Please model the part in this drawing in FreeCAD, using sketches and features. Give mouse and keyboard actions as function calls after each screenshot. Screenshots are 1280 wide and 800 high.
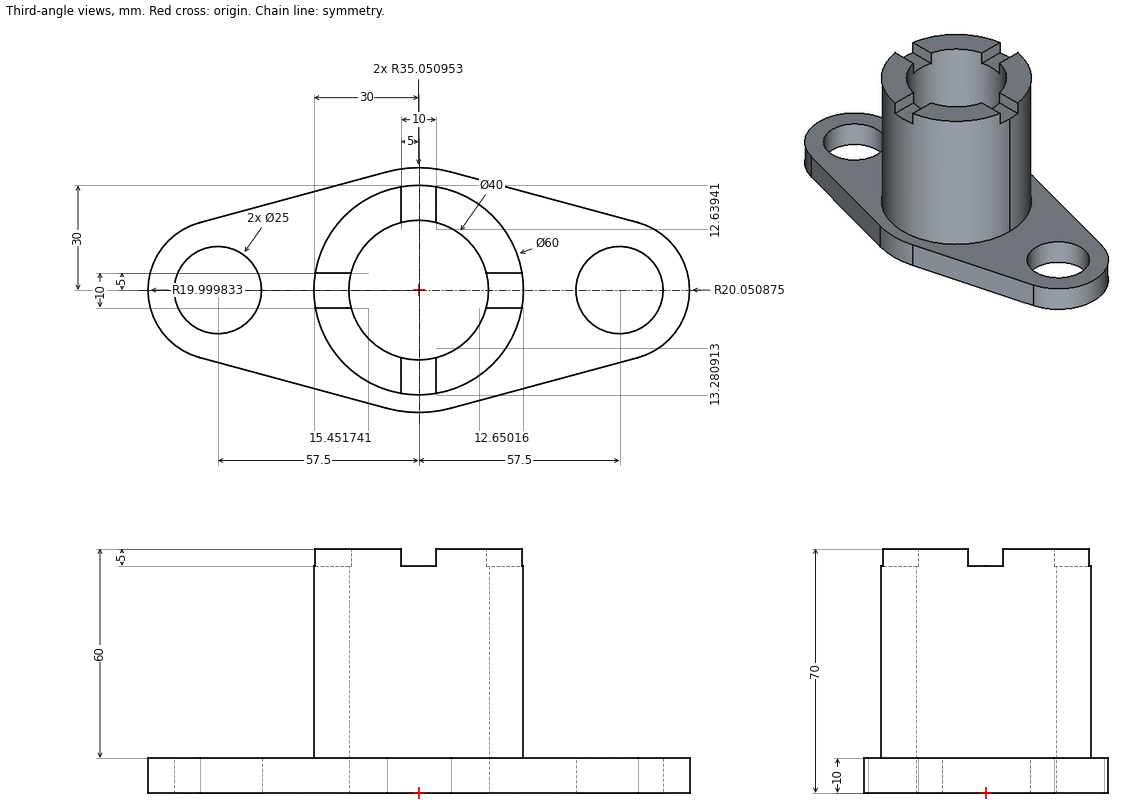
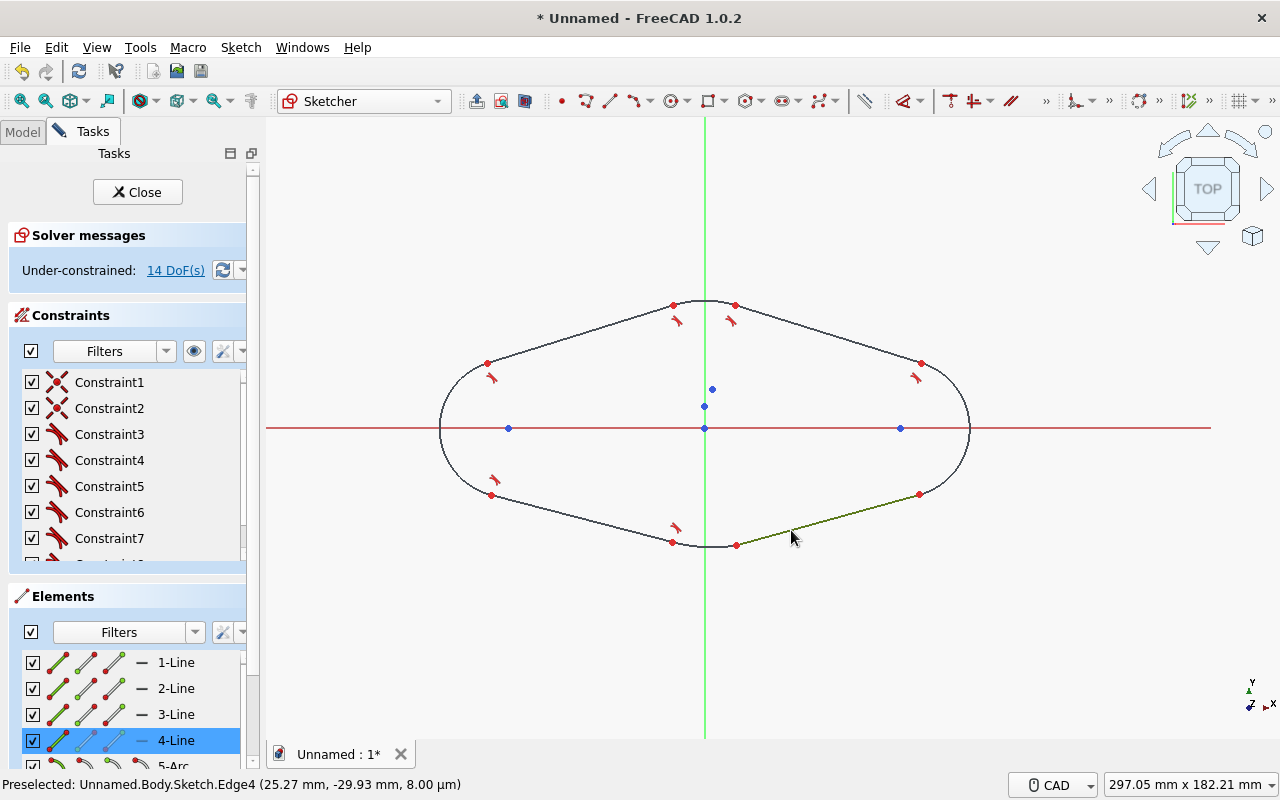
click(692, 546)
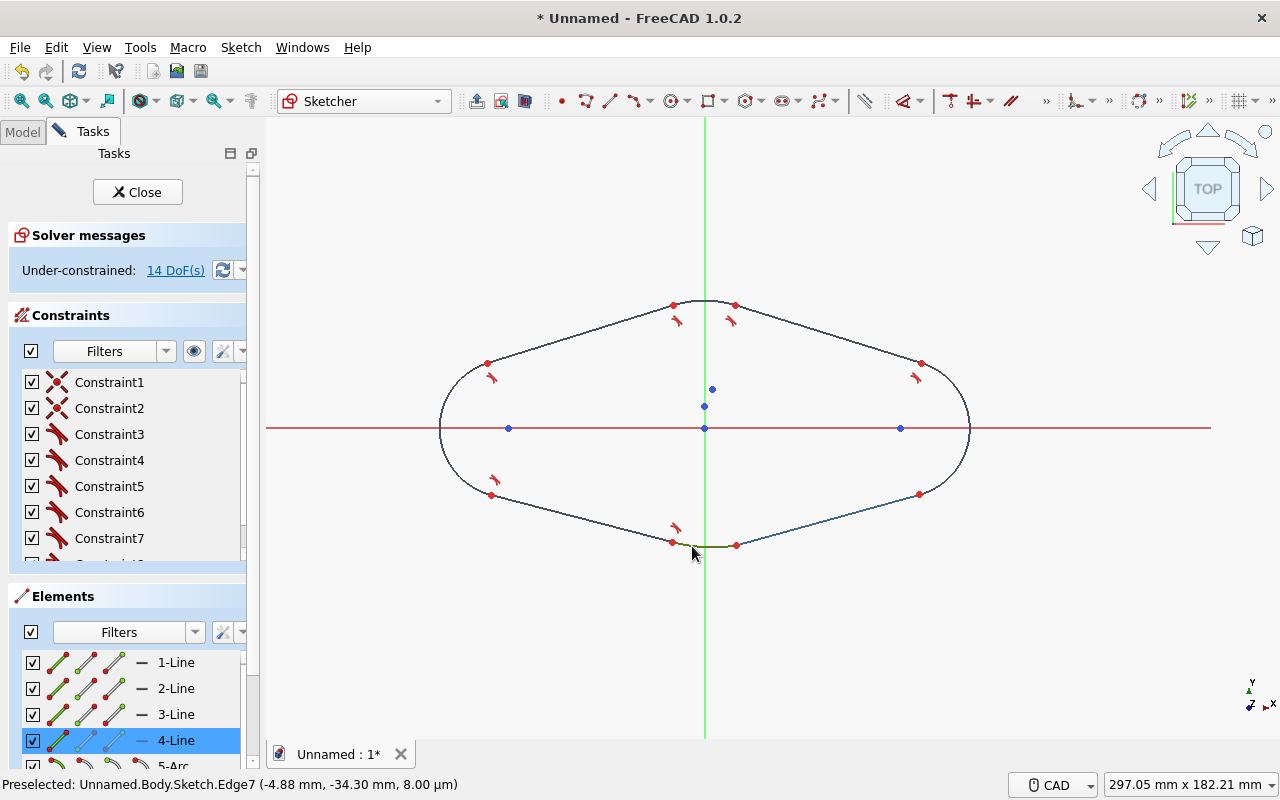
key(t)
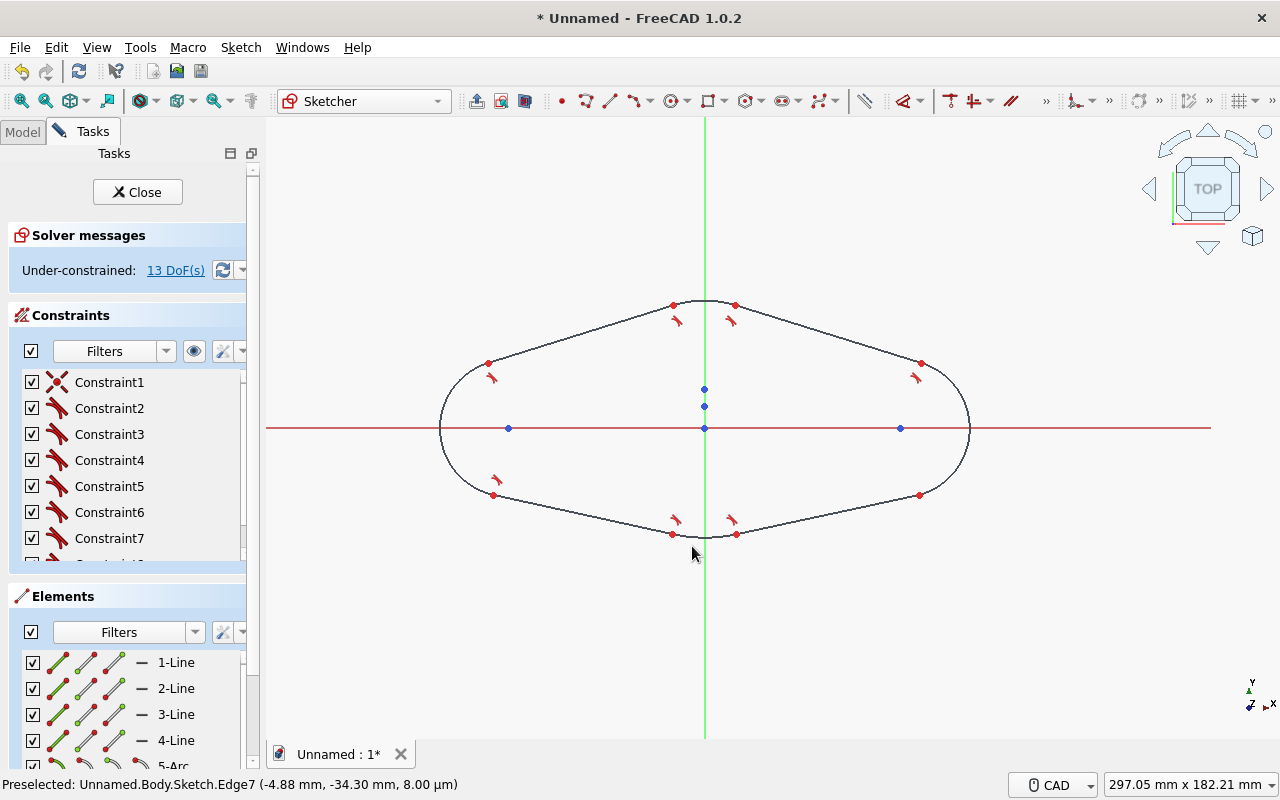
click(791, 523)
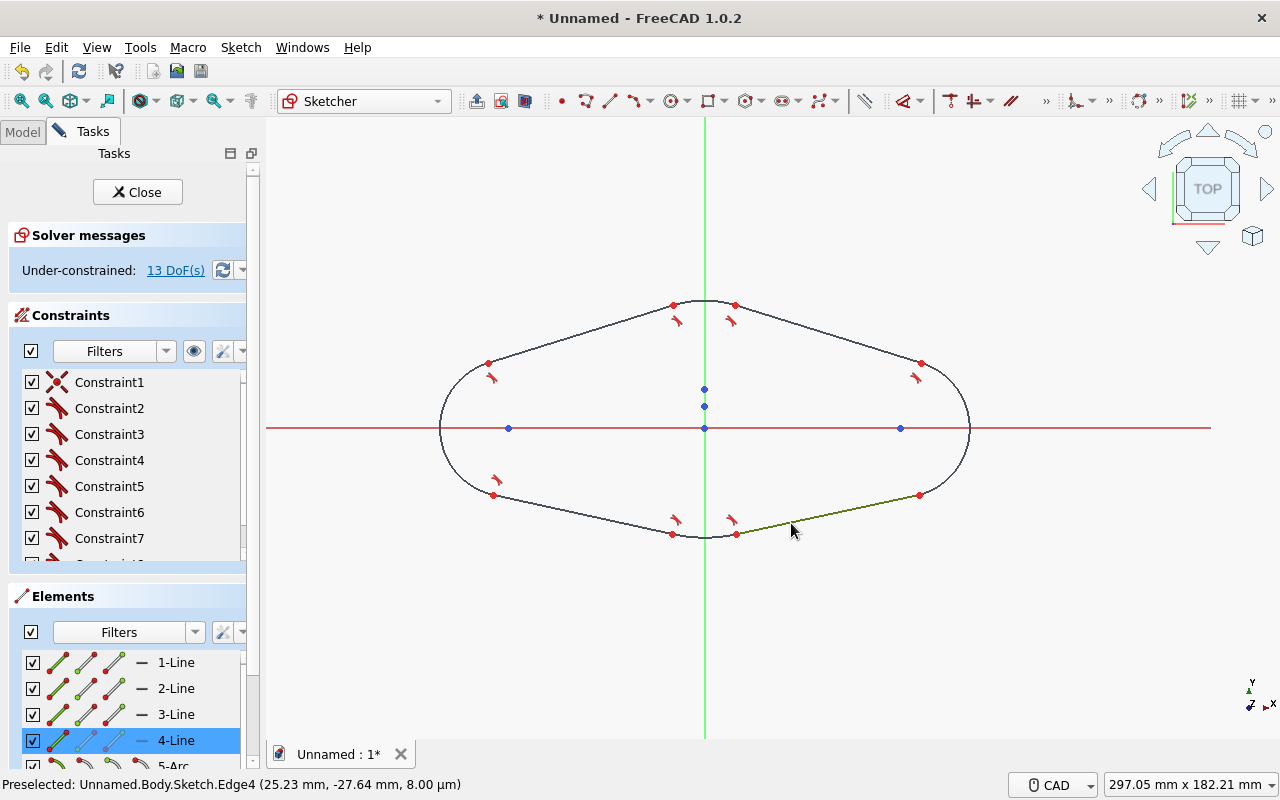
click(960, 464)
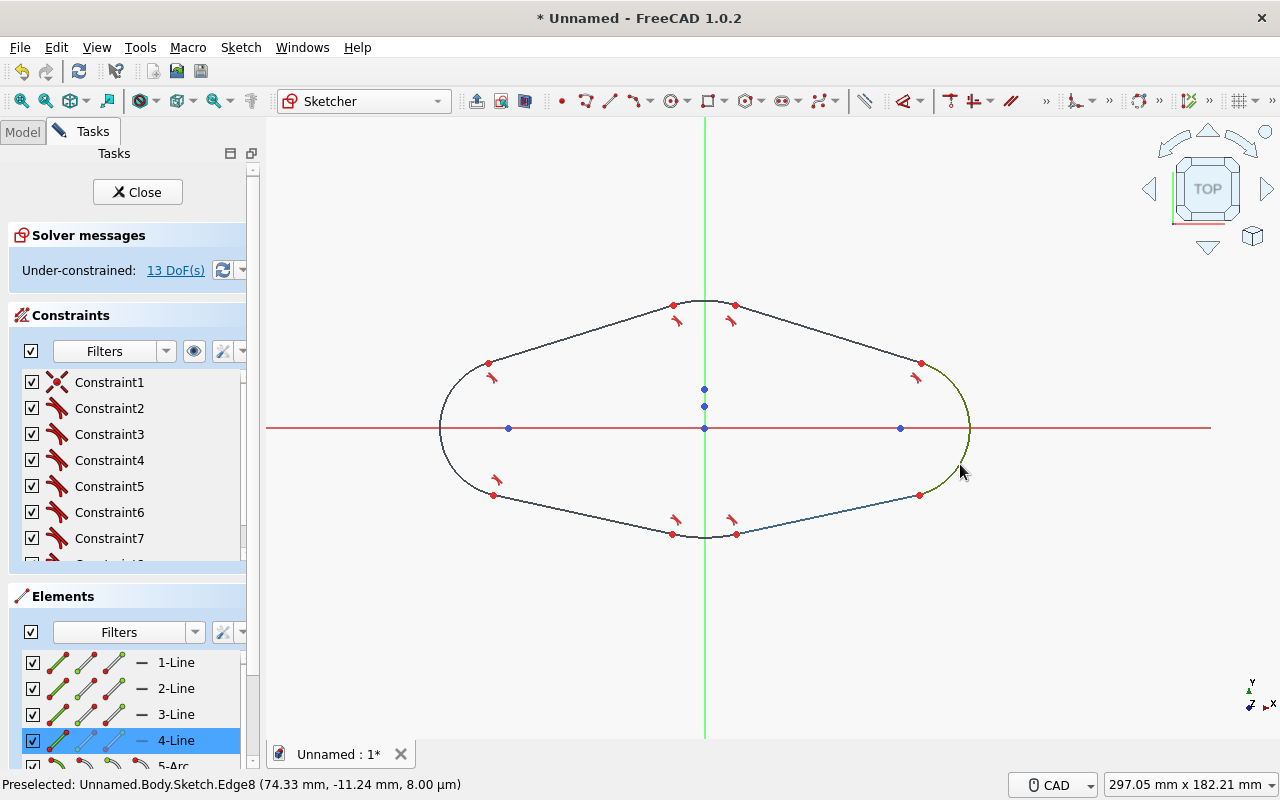
key(t)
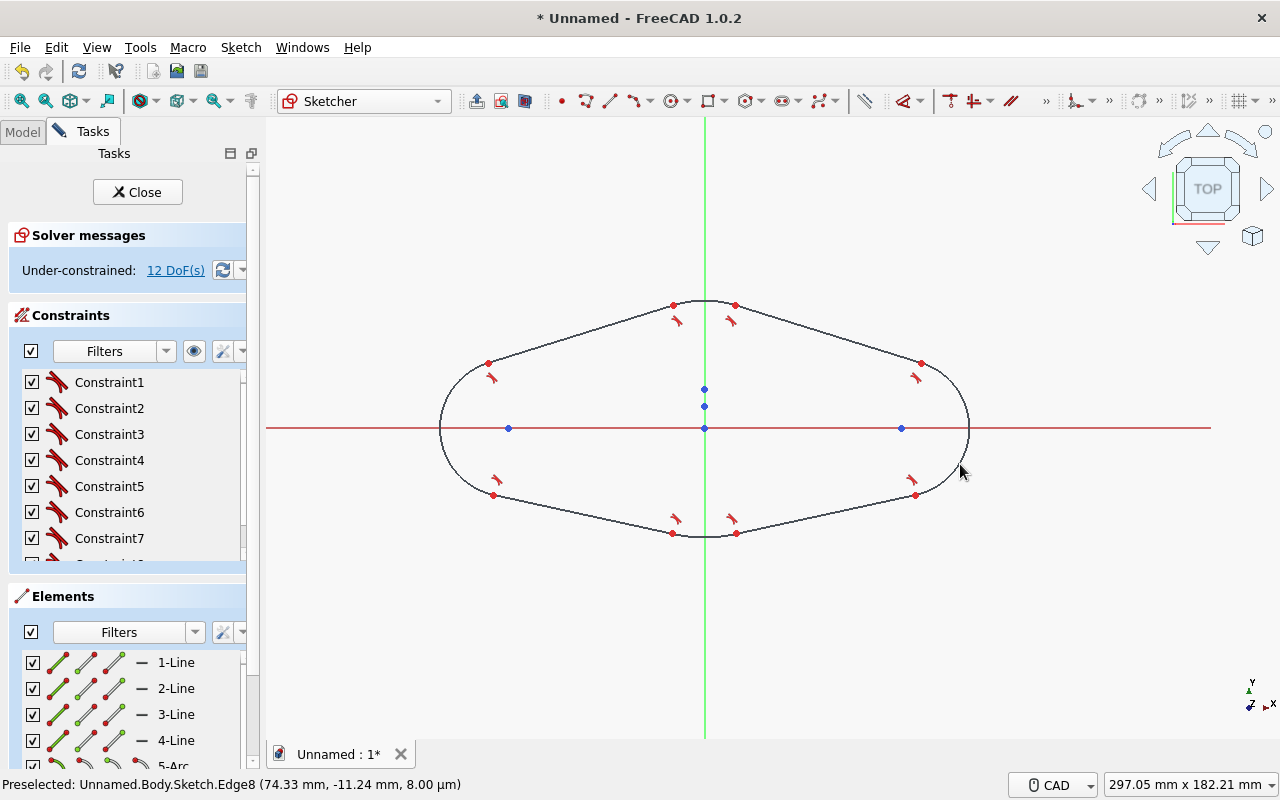
click(717, 301)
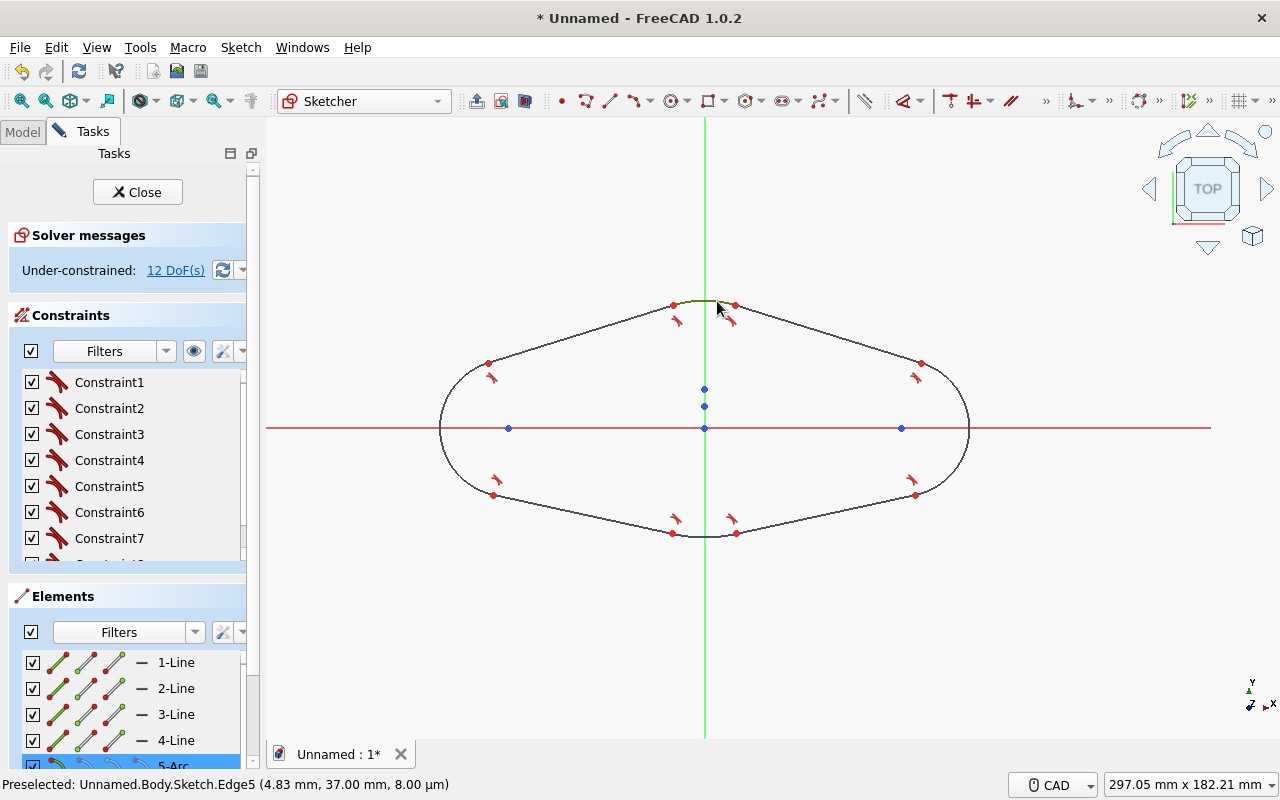
click(692, 537)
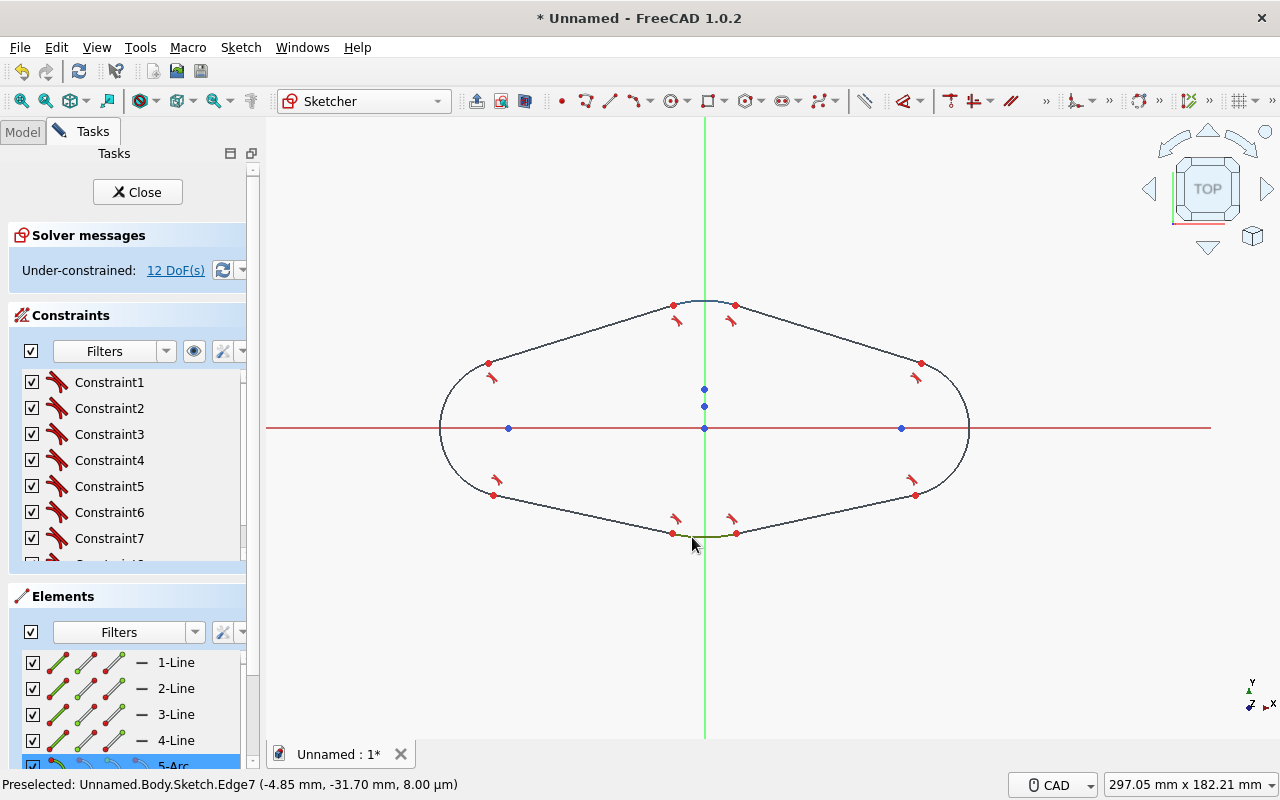
key(c)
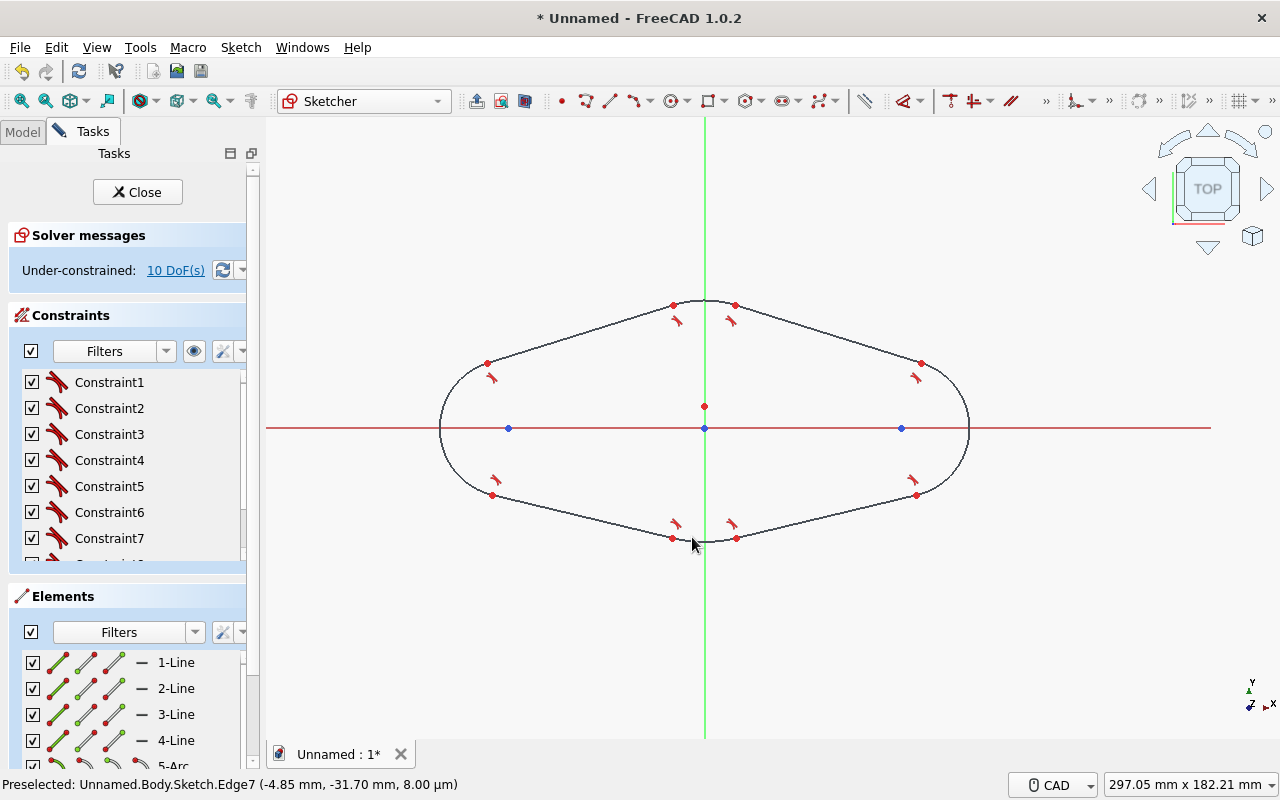
drag(695, 396, 715, 438)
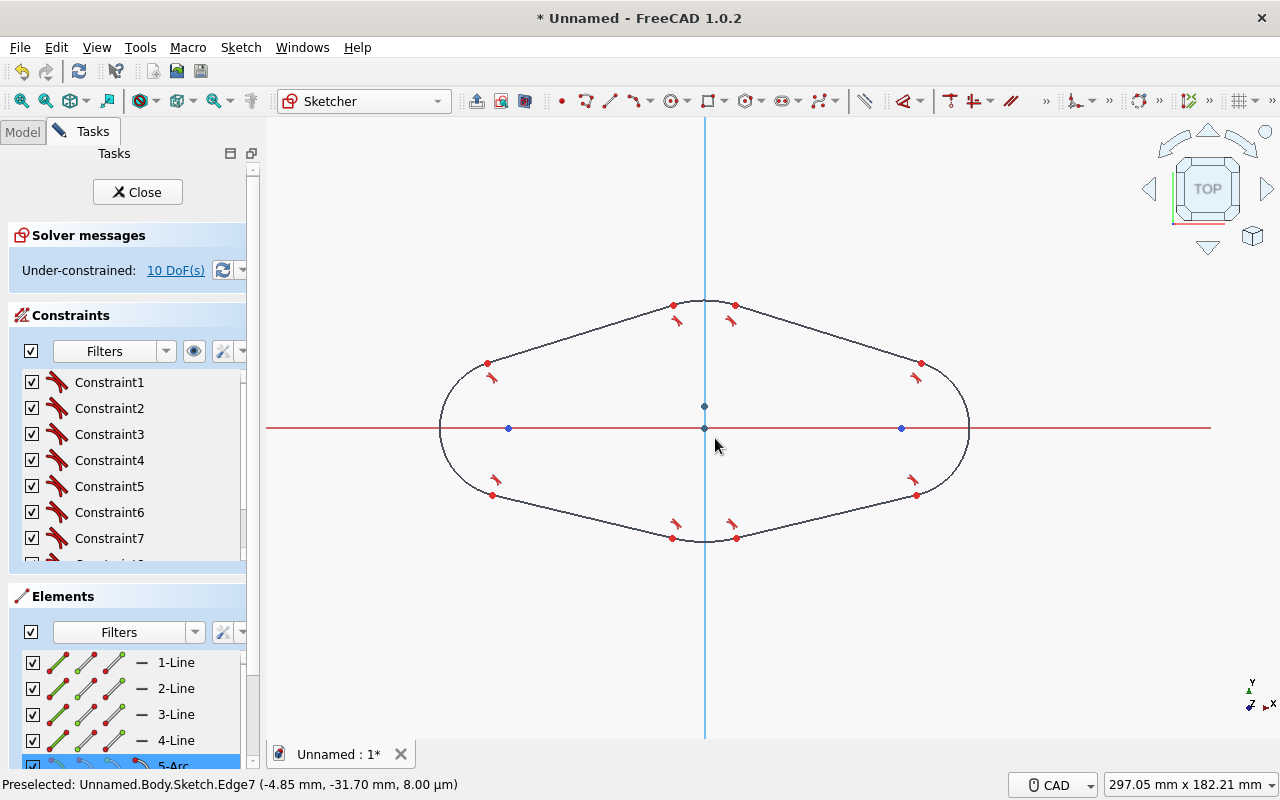
key(c)